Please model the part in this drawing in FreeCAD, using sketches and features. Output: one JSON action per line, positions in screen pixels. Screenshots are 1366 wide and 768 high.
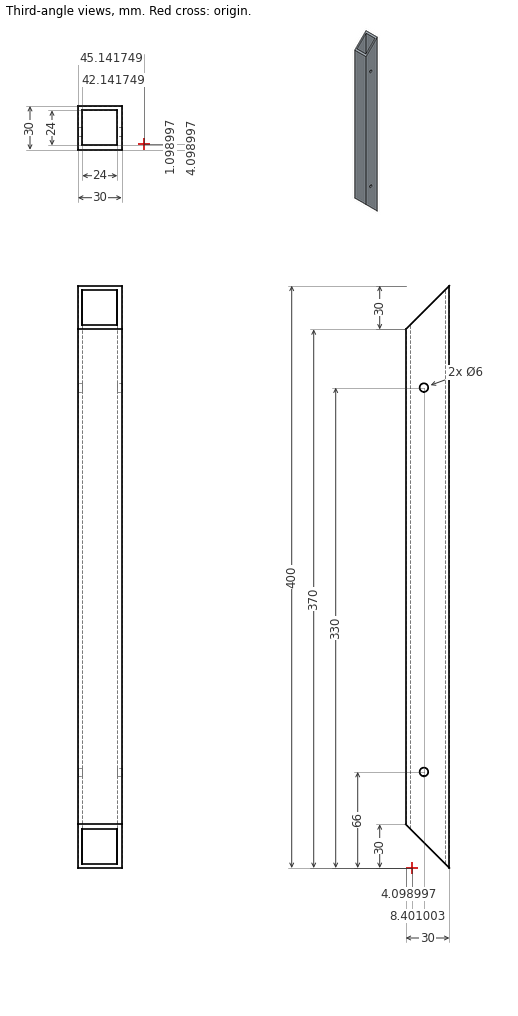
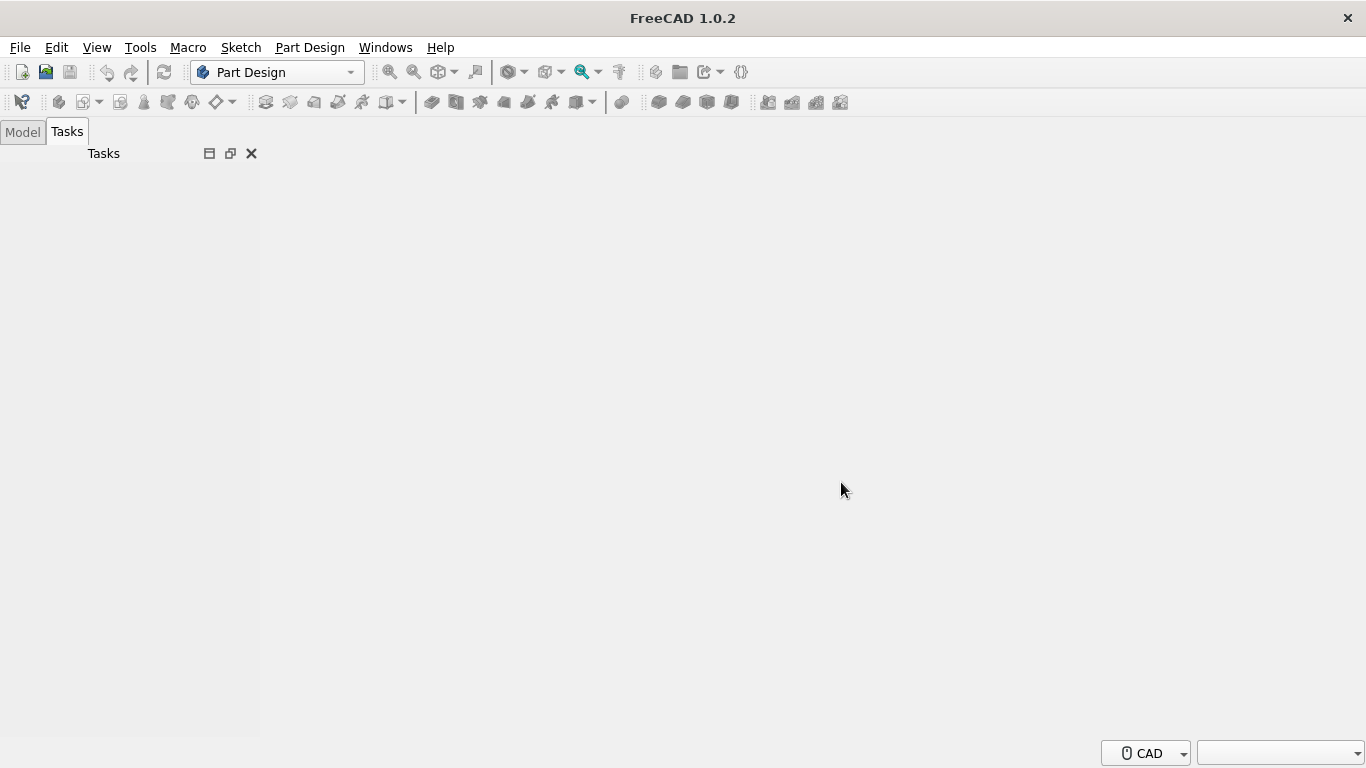
{"action": "left_click", "coordinate": [22, 72]}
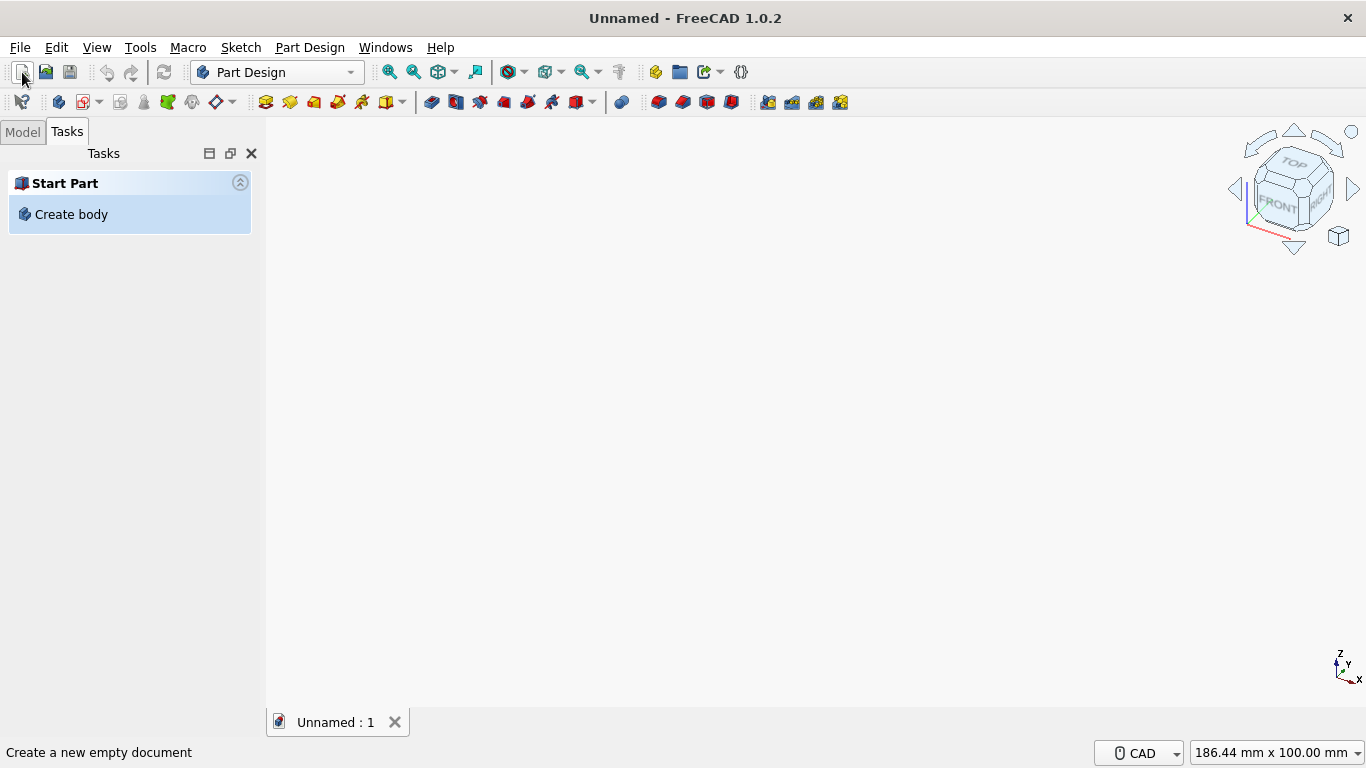
{"action": "left_click", "coordinate": [84, 102]}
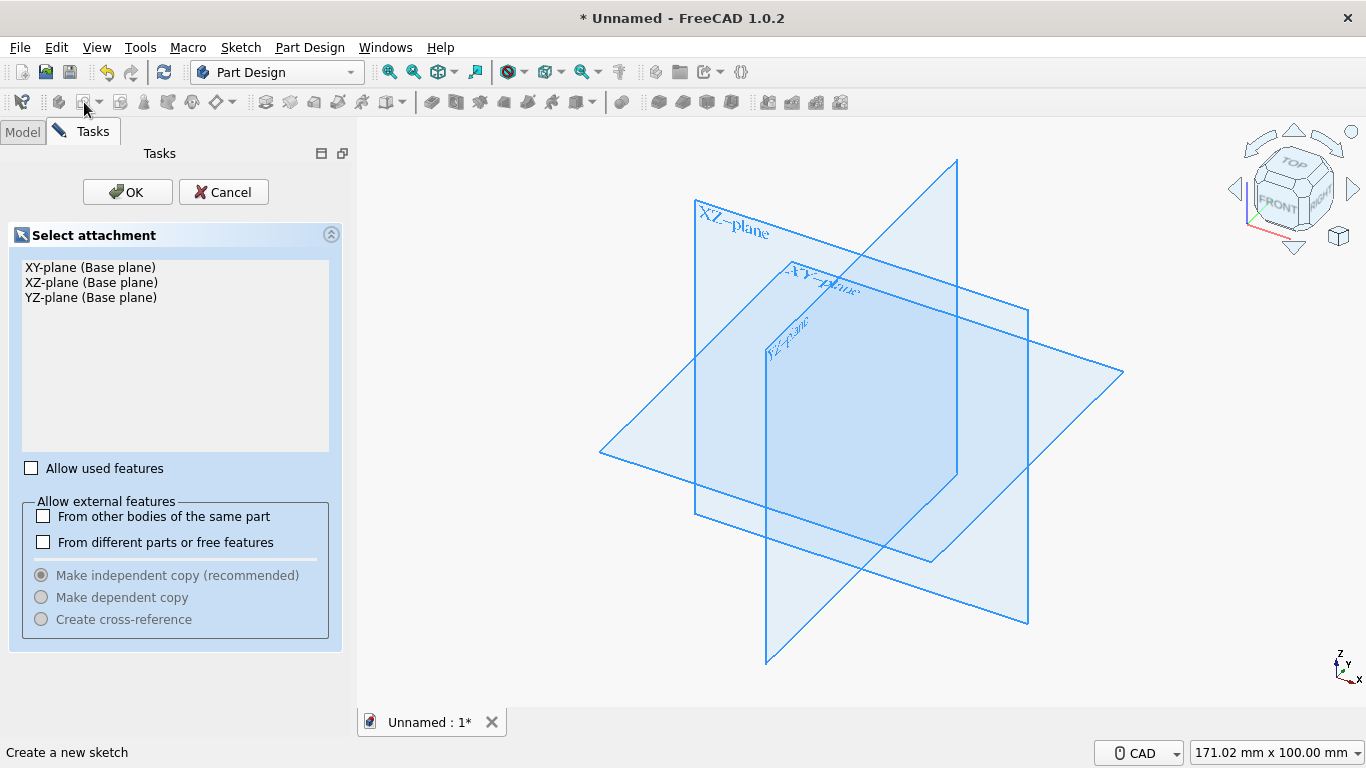
{"action": "left_click", "coordinate": [82, 268]}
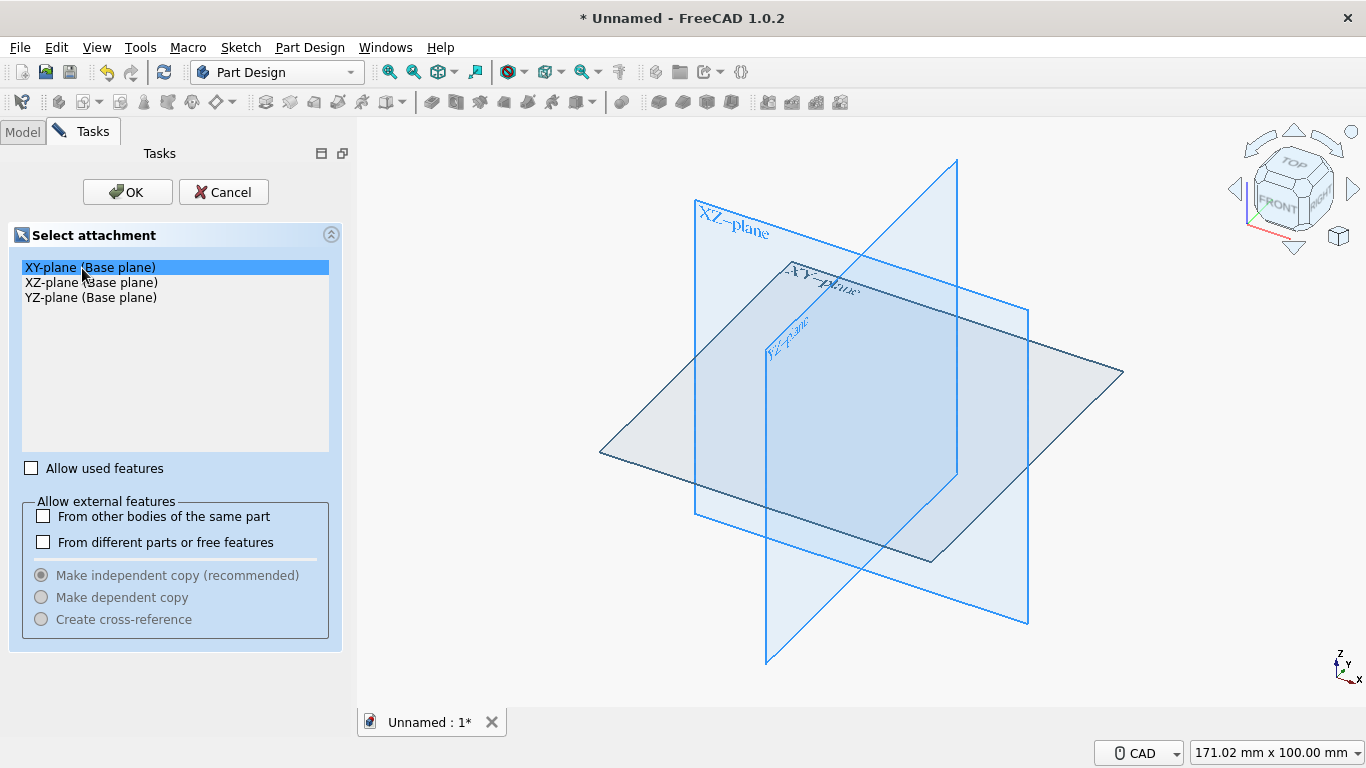
{"action": "left_click", "coordinate": [128, 192]}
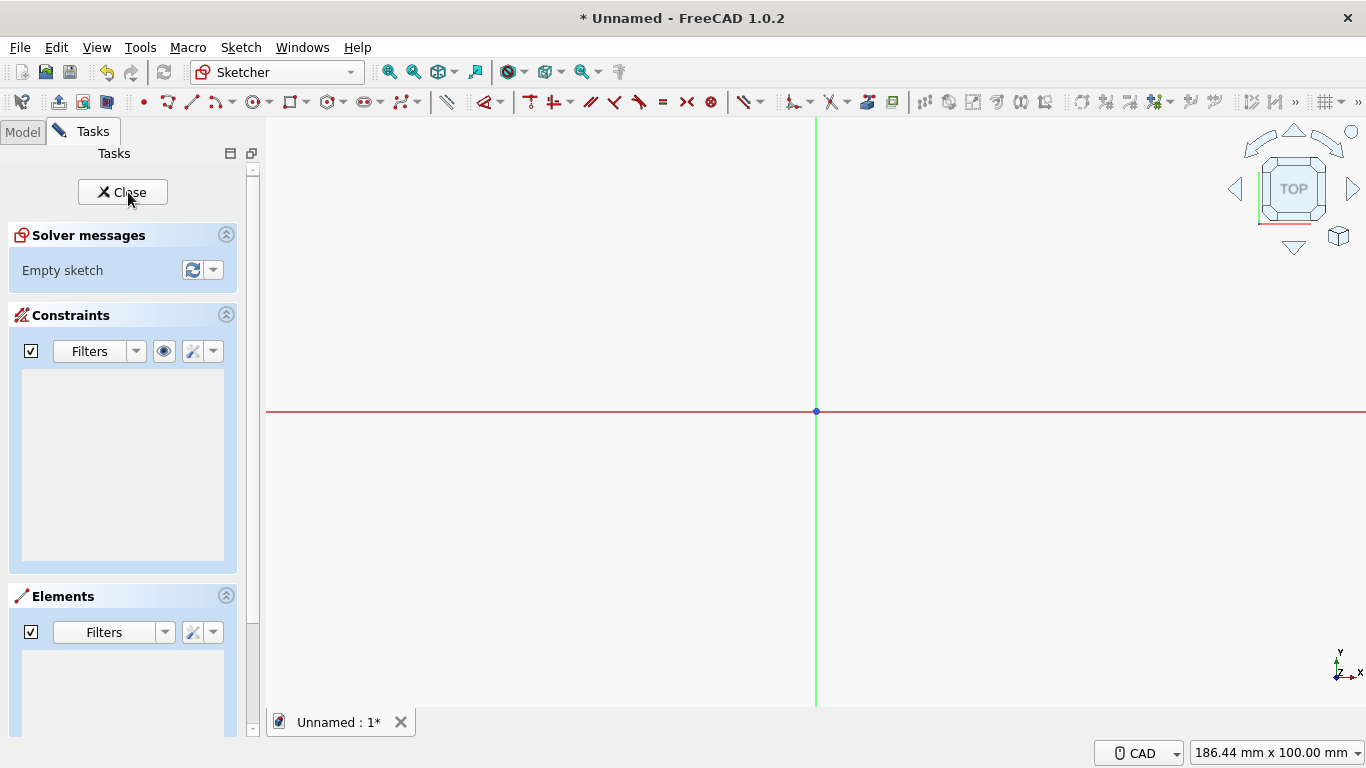
{"action": "scroll", "coordinate": [630, 295], "scroll_direction": "up", "scroll_amount": 4}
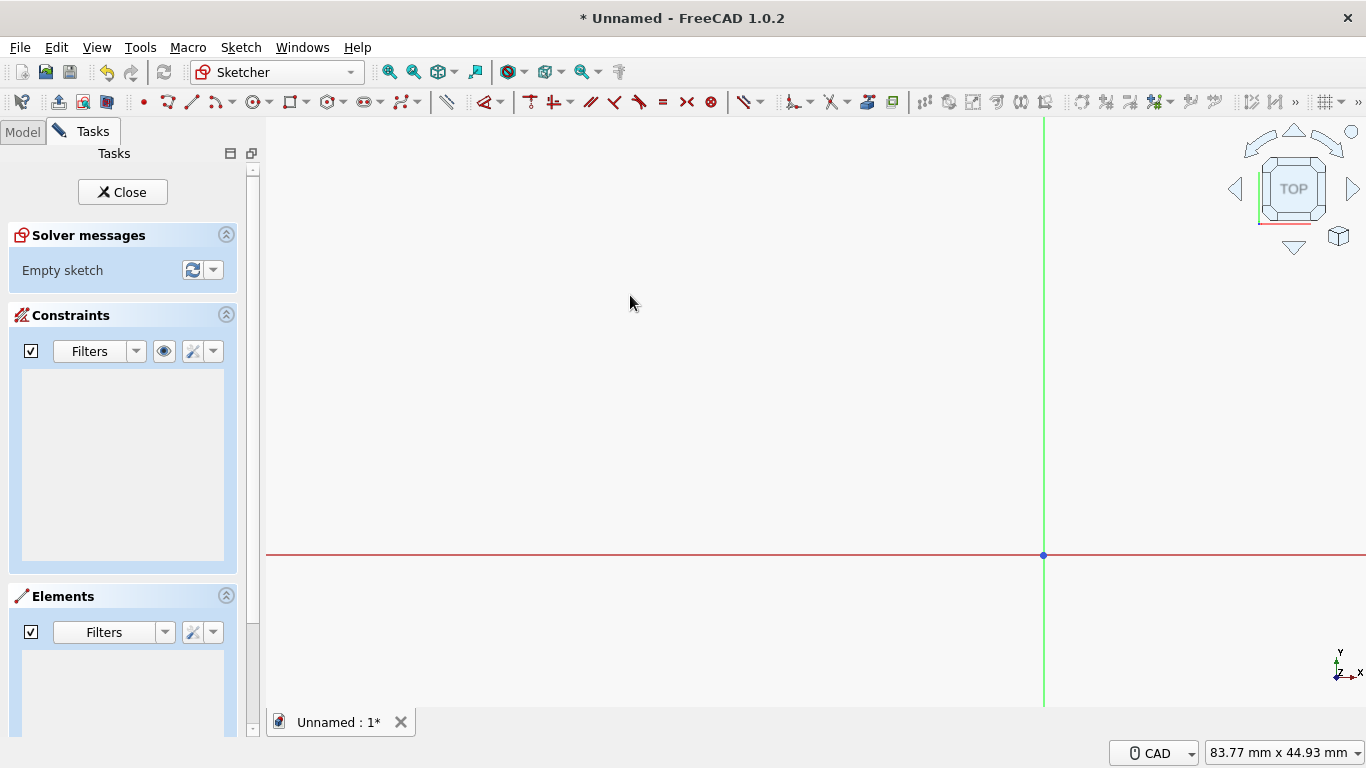
{"action": "left_click", "coordinate": [290, 102]}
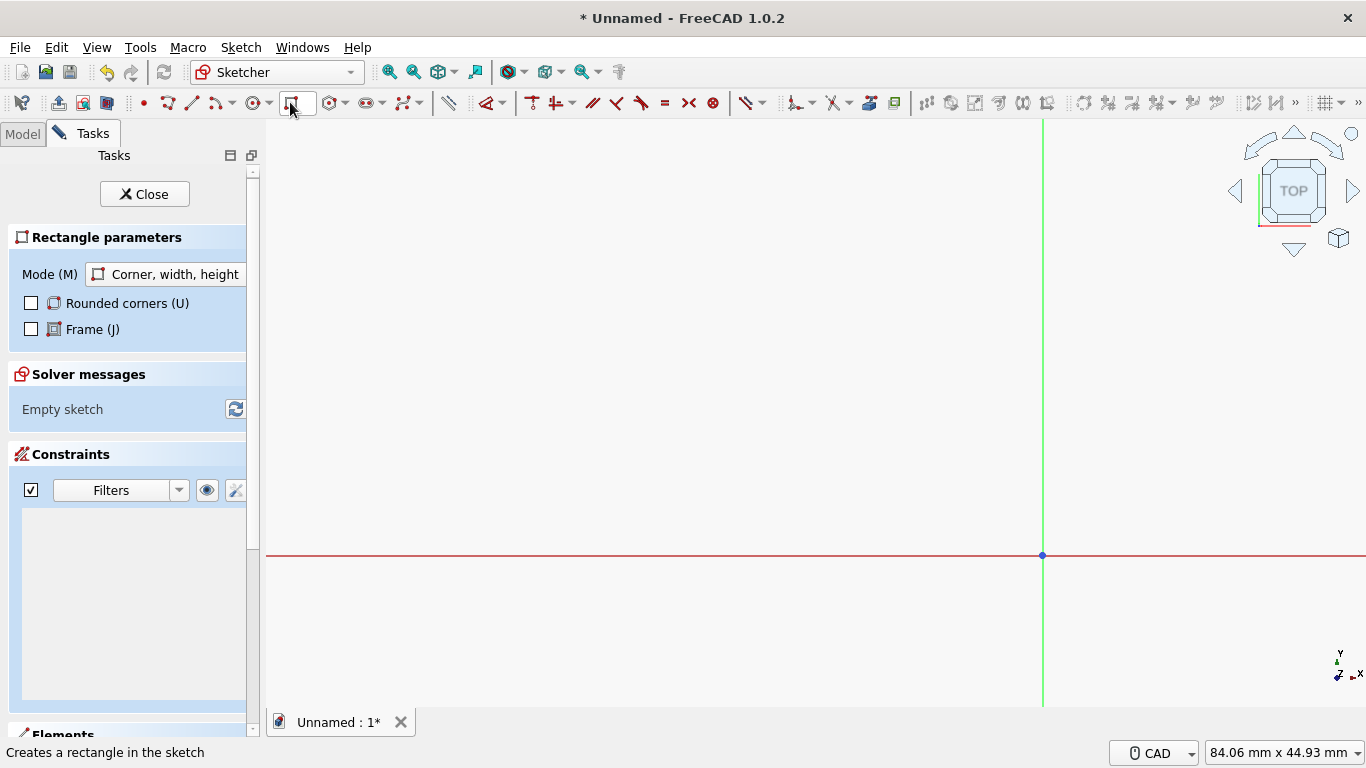
{"action": "left_click", "coordinate": [452, 217]}
{"action": "left_click", "coordinate": [845, 609]}
{"action": "key", "text": "Escape"}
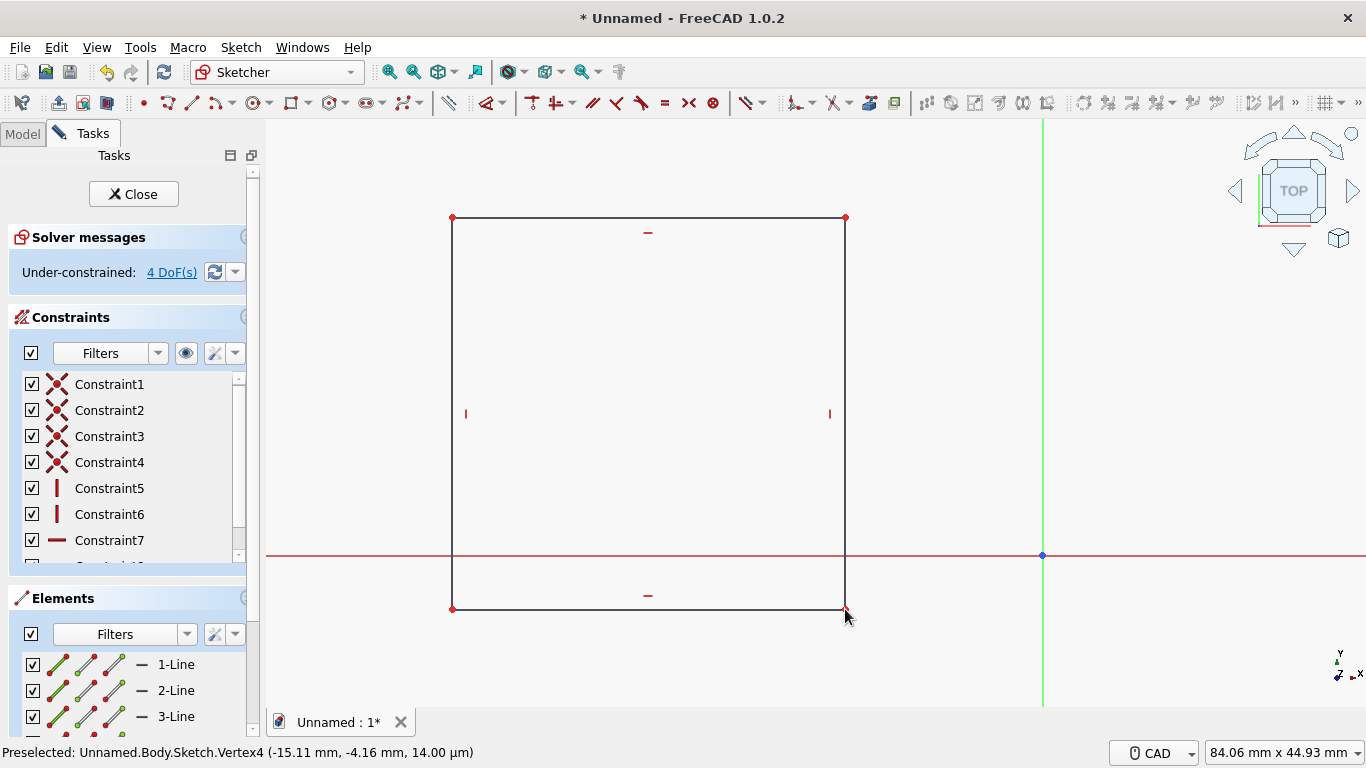
{"action": "key", "text": "d"}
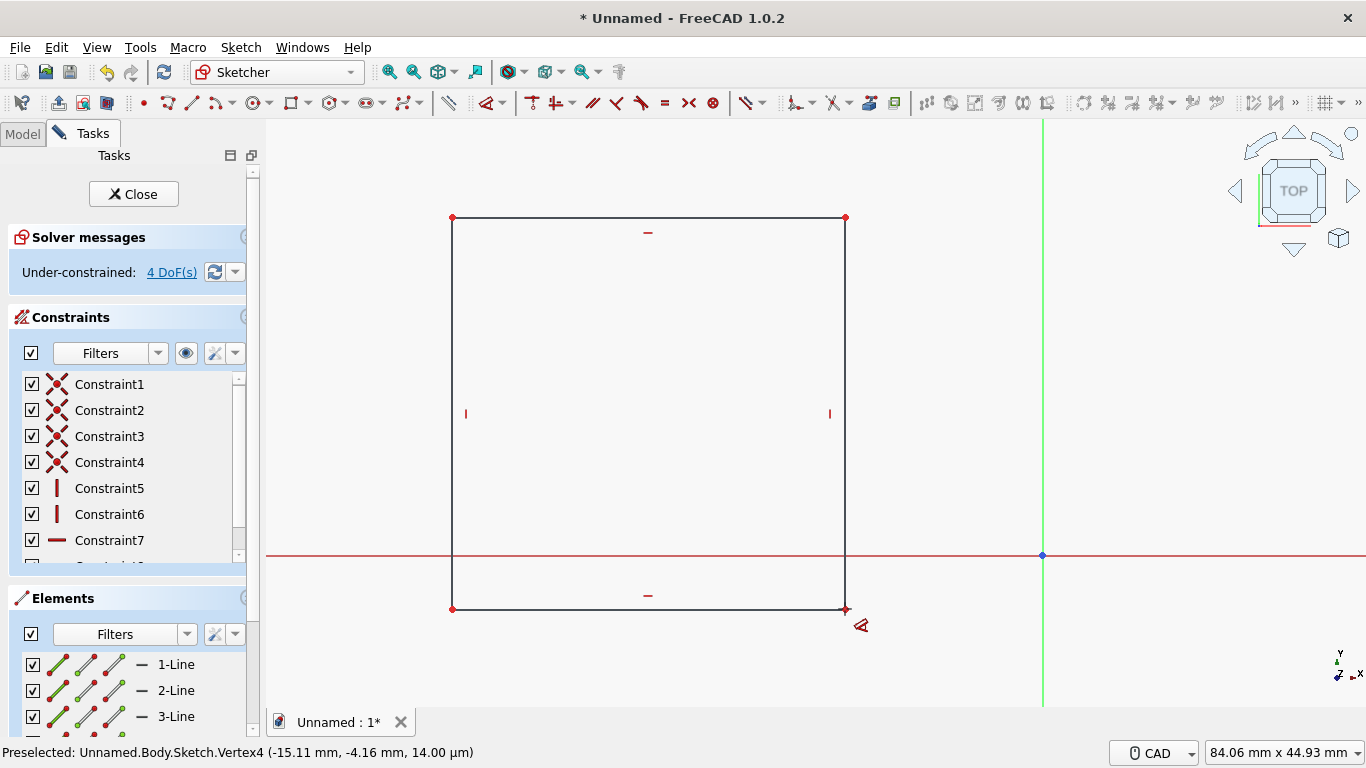
{"action": "left_click", "coordinate": [452, 336]}
{"action": "left_click", "coordinate": [418, 414]}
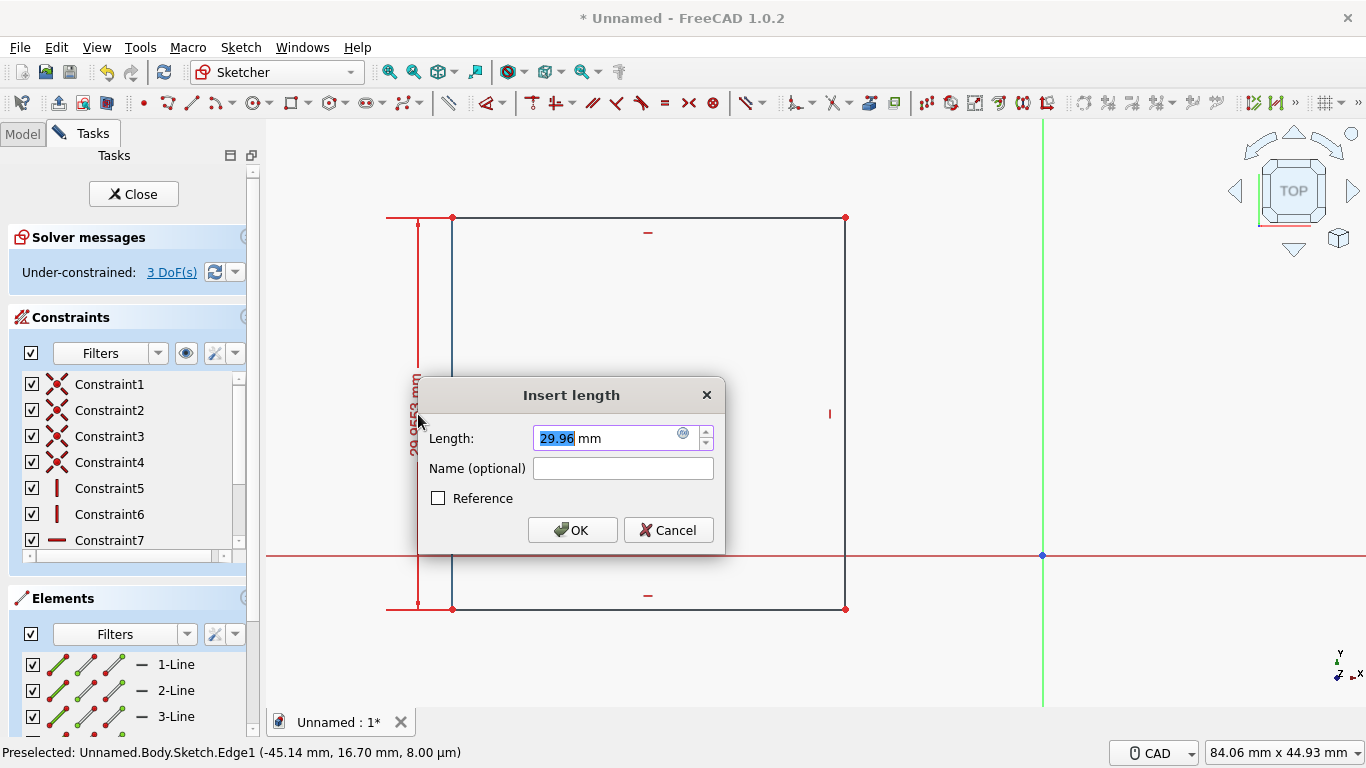
{"action": "type", "text": "30"}
{"action": "key", "text": "Return"}